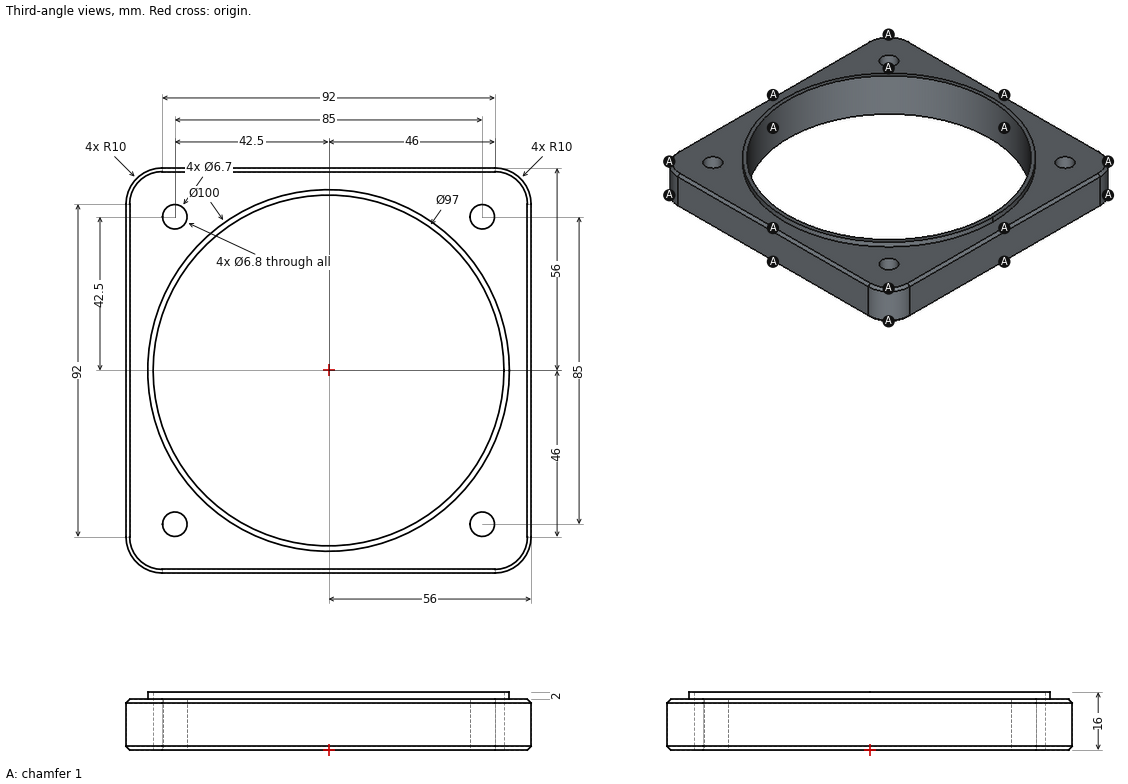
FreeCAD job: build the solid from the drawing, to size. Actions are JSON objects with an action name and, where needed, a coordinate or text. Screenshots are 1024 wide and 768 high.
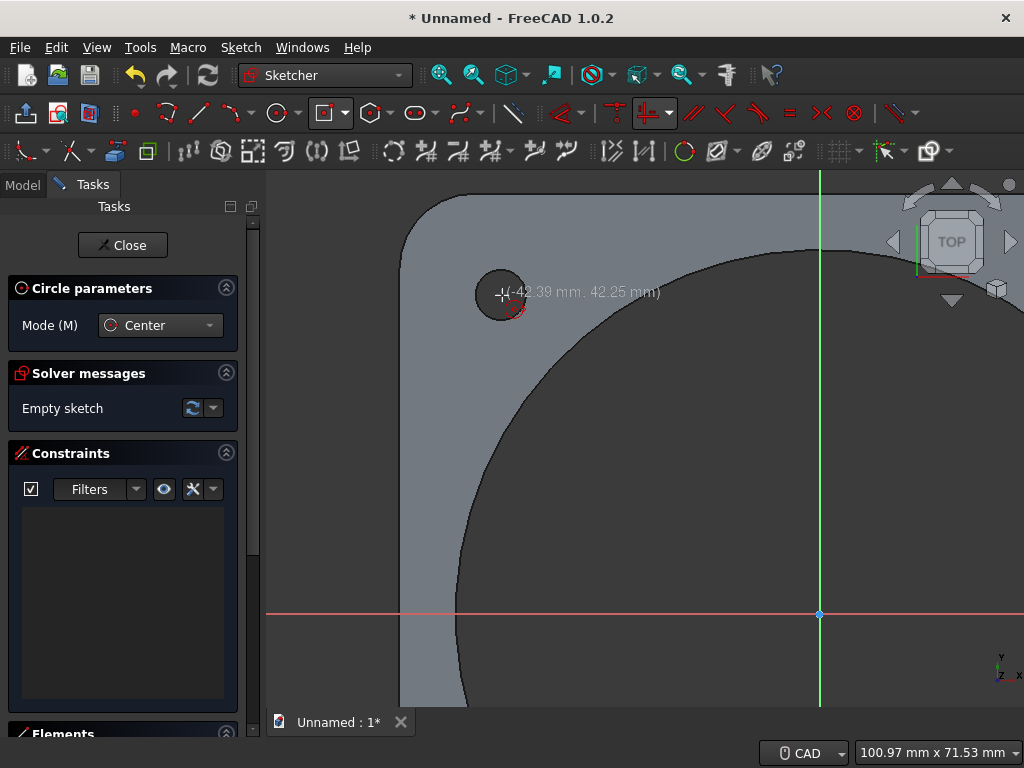
{"action": "left_click", "coordinate": [501, 295]}
{"action": "mouse_move", "coordinate": [519, 277]}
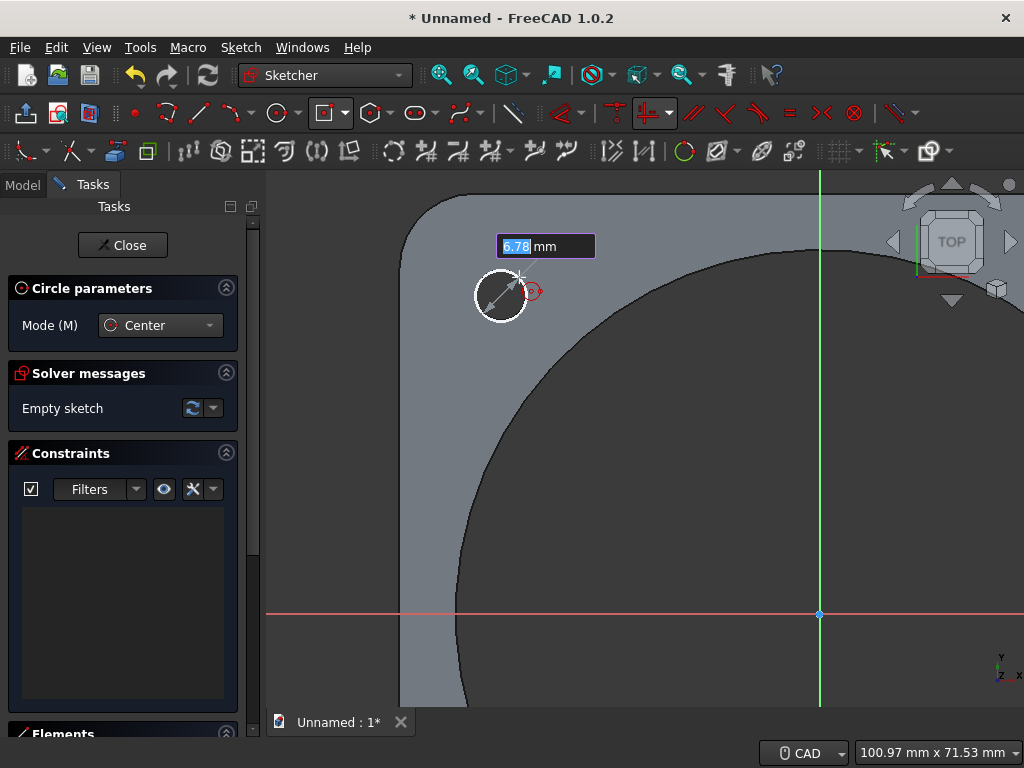
{"action": "type", "text": "6.8"}
{"action": "key", "text": "Return"}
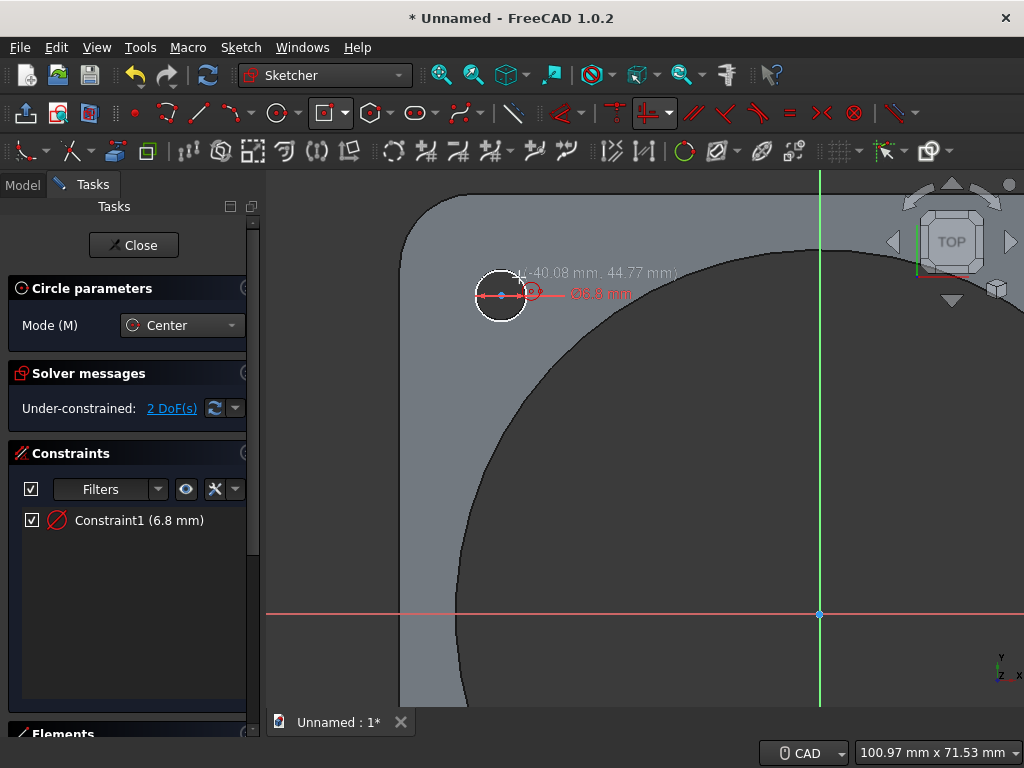
{"action": "scroll", "coordinate": [378, 295], "scroll_direction": "down", "scroll_amount": 4}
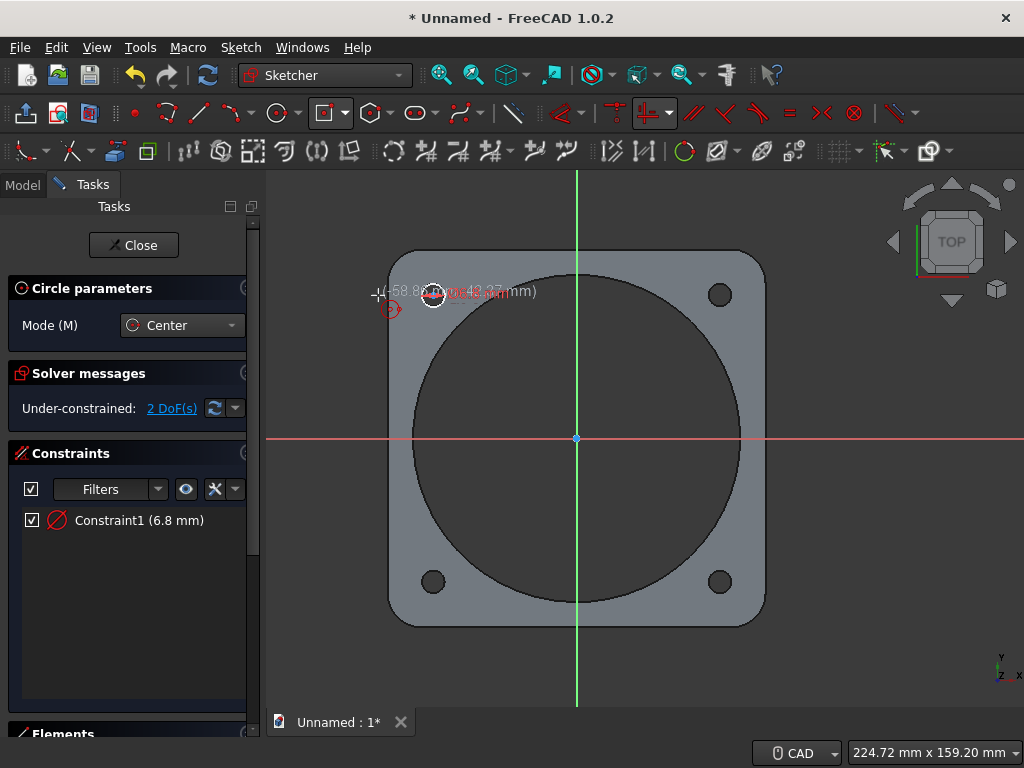
{"action": "scroll", "coordinate": [720, 295], "scroll_direction": "up", "scroll_amount": 4}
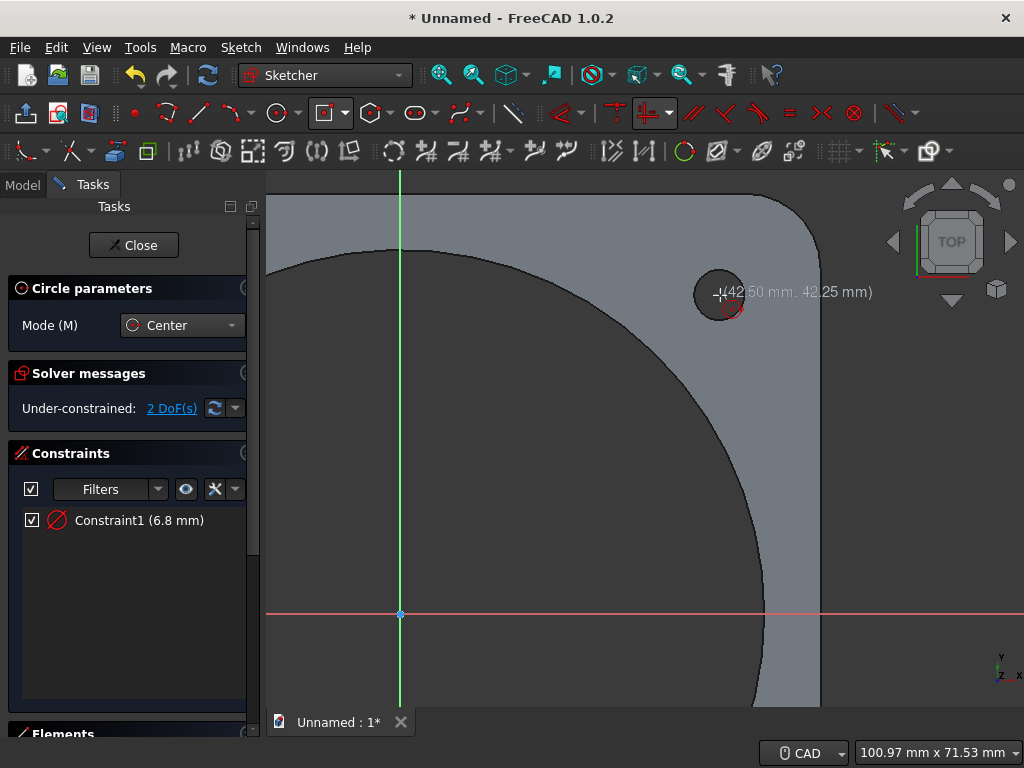
{"action": "left_click", "coordinate": [719, 295]}
{"action": "mouse_move", "coordinate": [737, 277]}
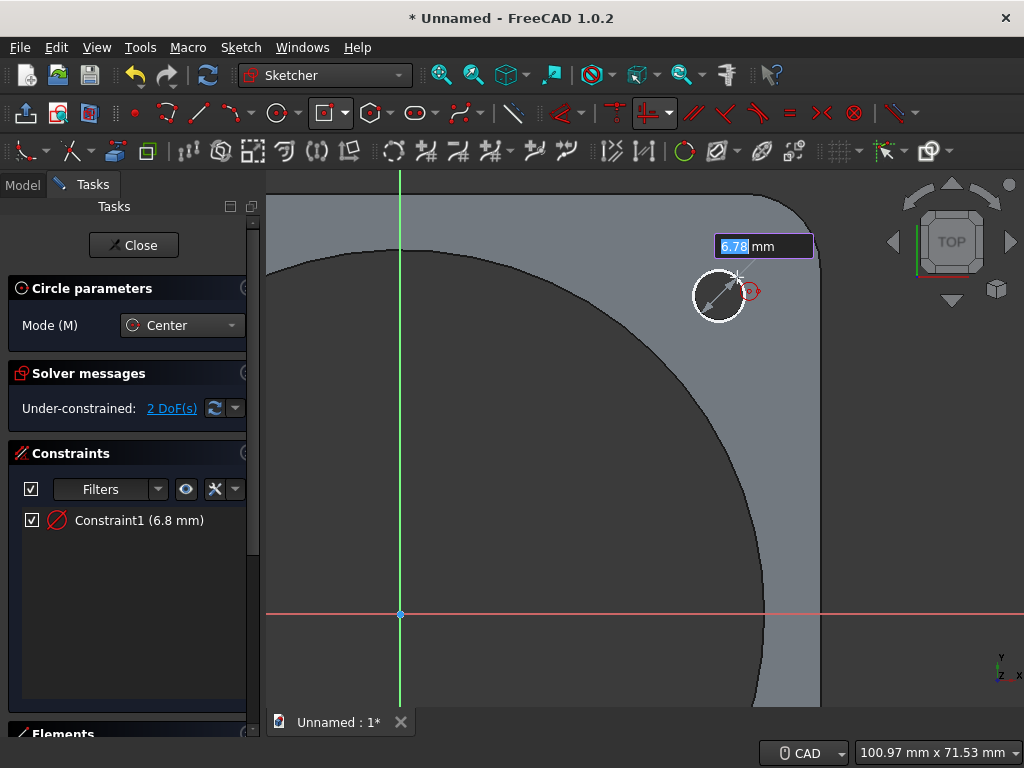
{"action": "type", "text": "6.8"}
{"action": "key", "text": "Return"}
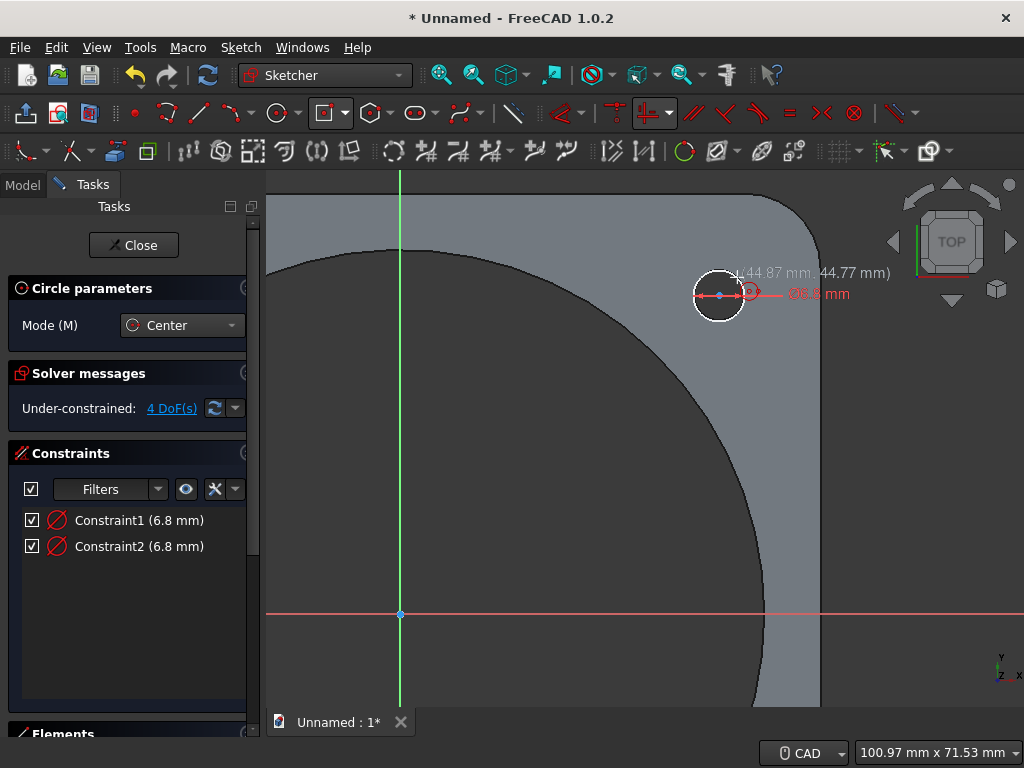
{"action": "scroll", "coordinate": [720, 295], "scroll_direction": "down", "scroll_amount": 4}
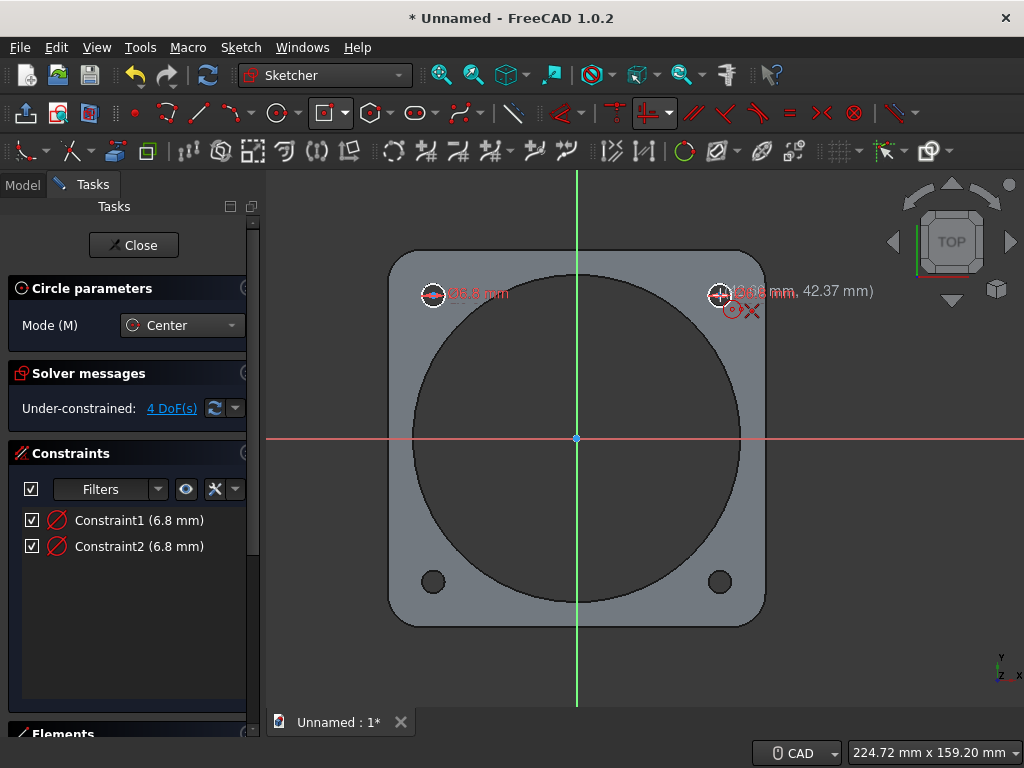
{"action": "scroll", "coordinate": [720, 582], "scroll_direction": "up", "scroll_amount": 4}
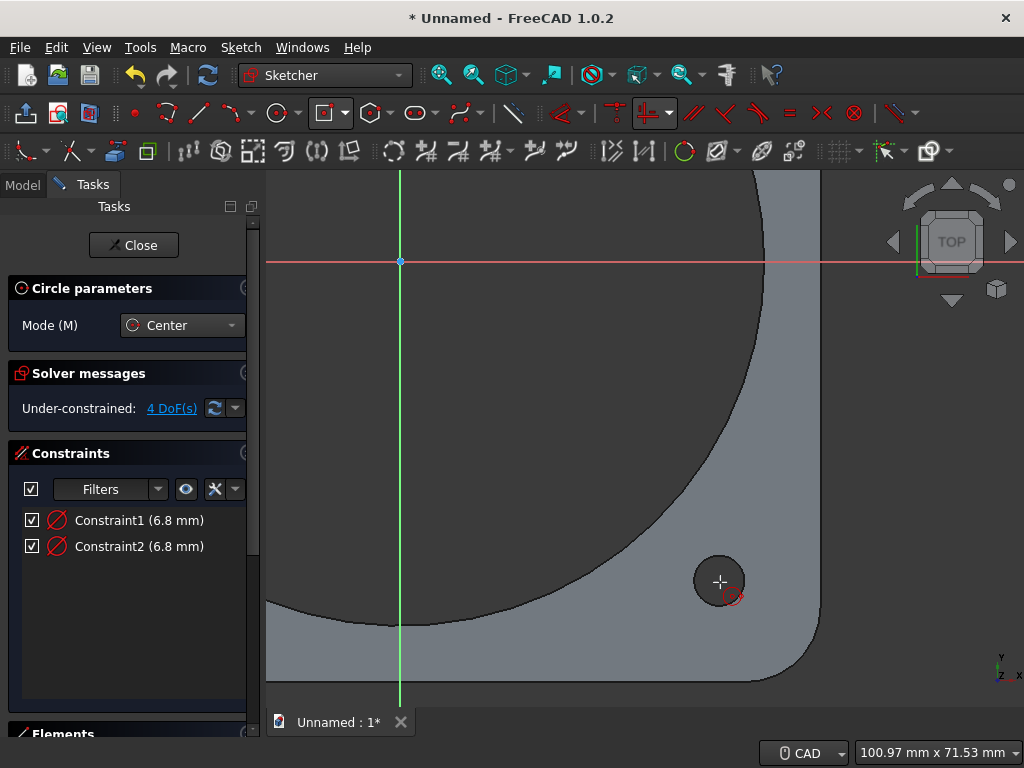
{"action": "left_click", "coordinate": [719, 581]}
{"action": "mouse_move", "coordinate": [737, 563]}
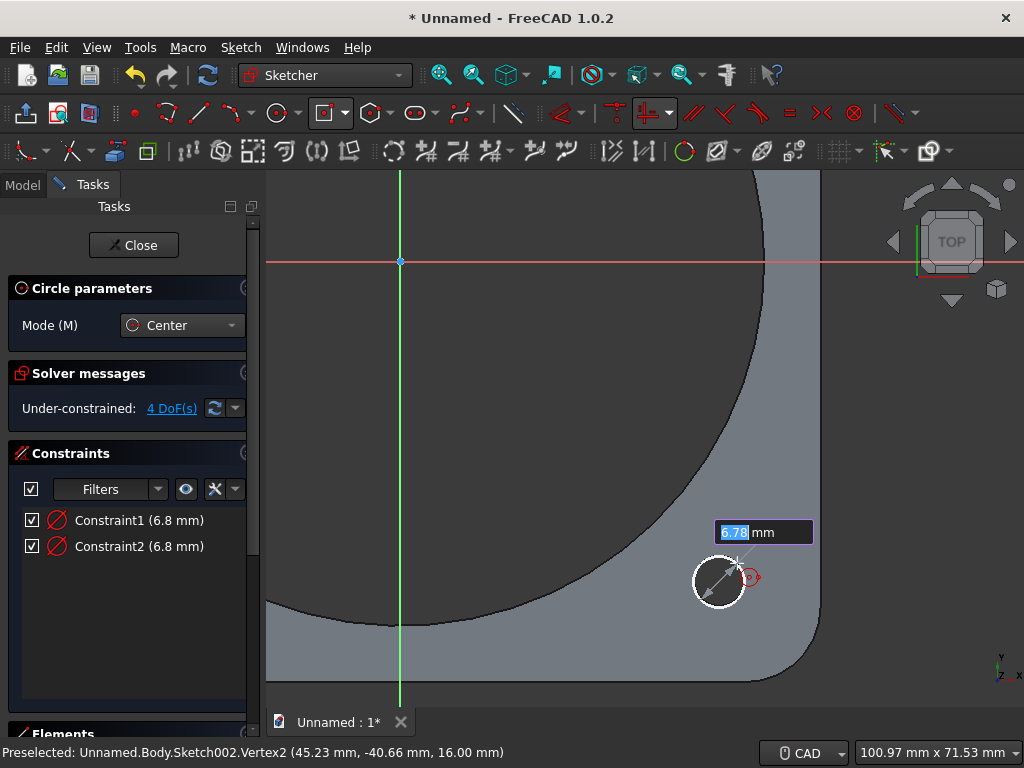
{"action": "type", "text": "6.8"}
{"action": "key", "text": "Return"}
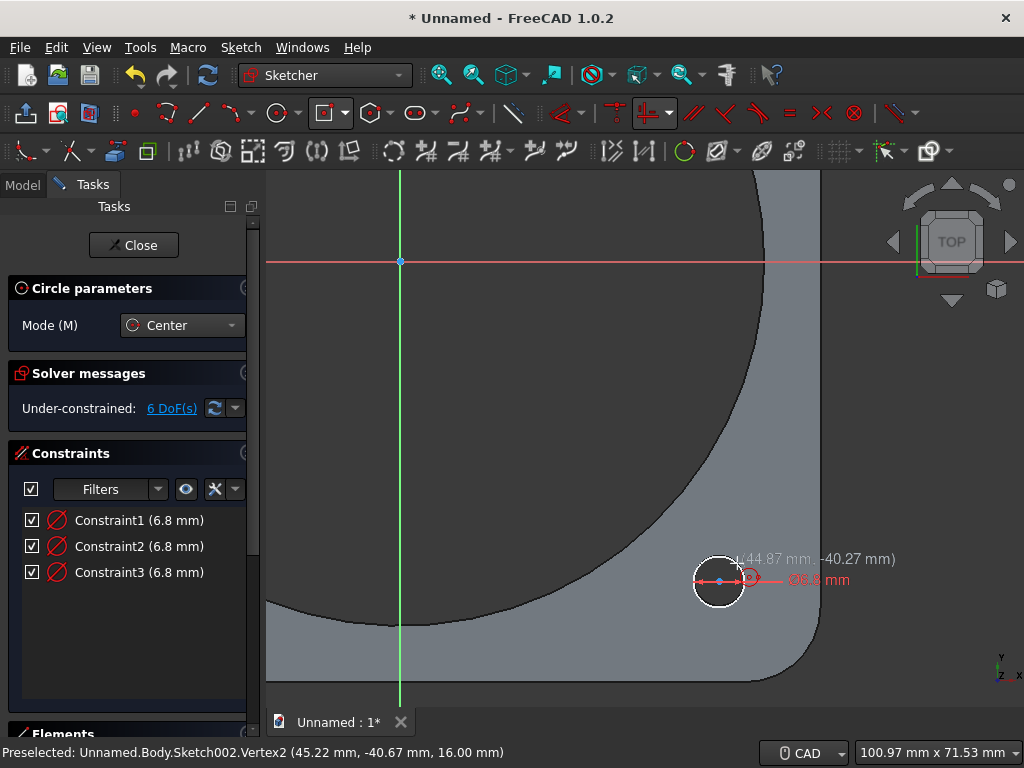
{"action": "scroll", "coordinate": [720, 583], "scroll_direction": "down", "scroll_amount": 4}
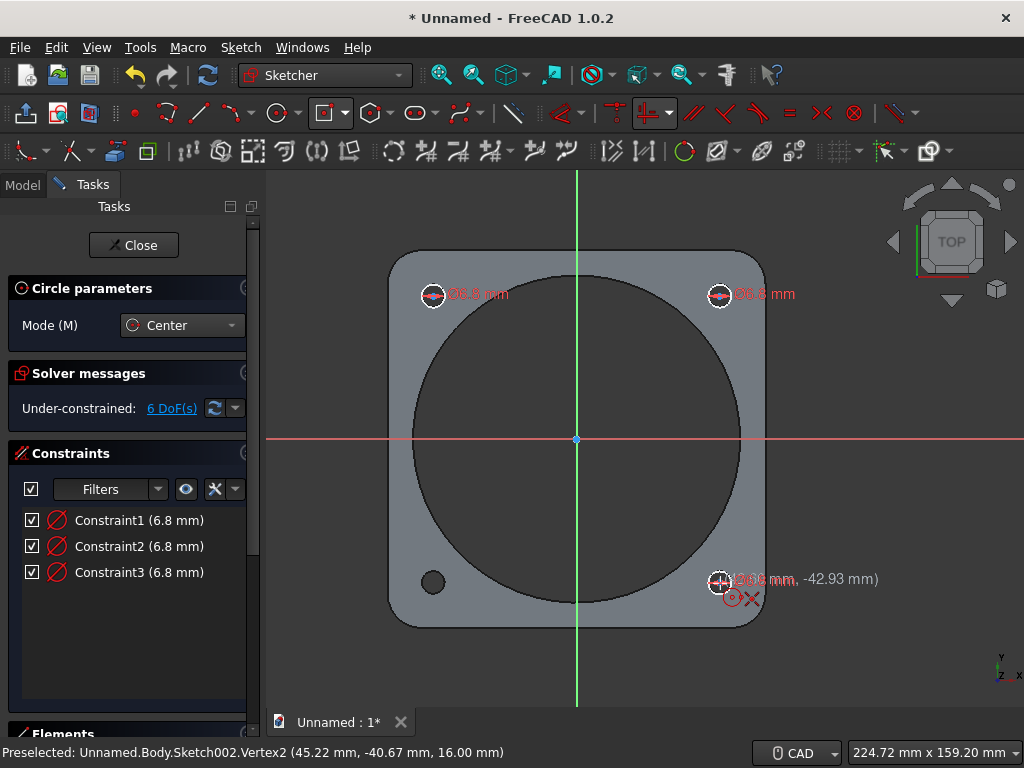
{"action": "scroll", "coordinate": [433, 582], "scroll_direction": "up", "scroll_amount": 4}